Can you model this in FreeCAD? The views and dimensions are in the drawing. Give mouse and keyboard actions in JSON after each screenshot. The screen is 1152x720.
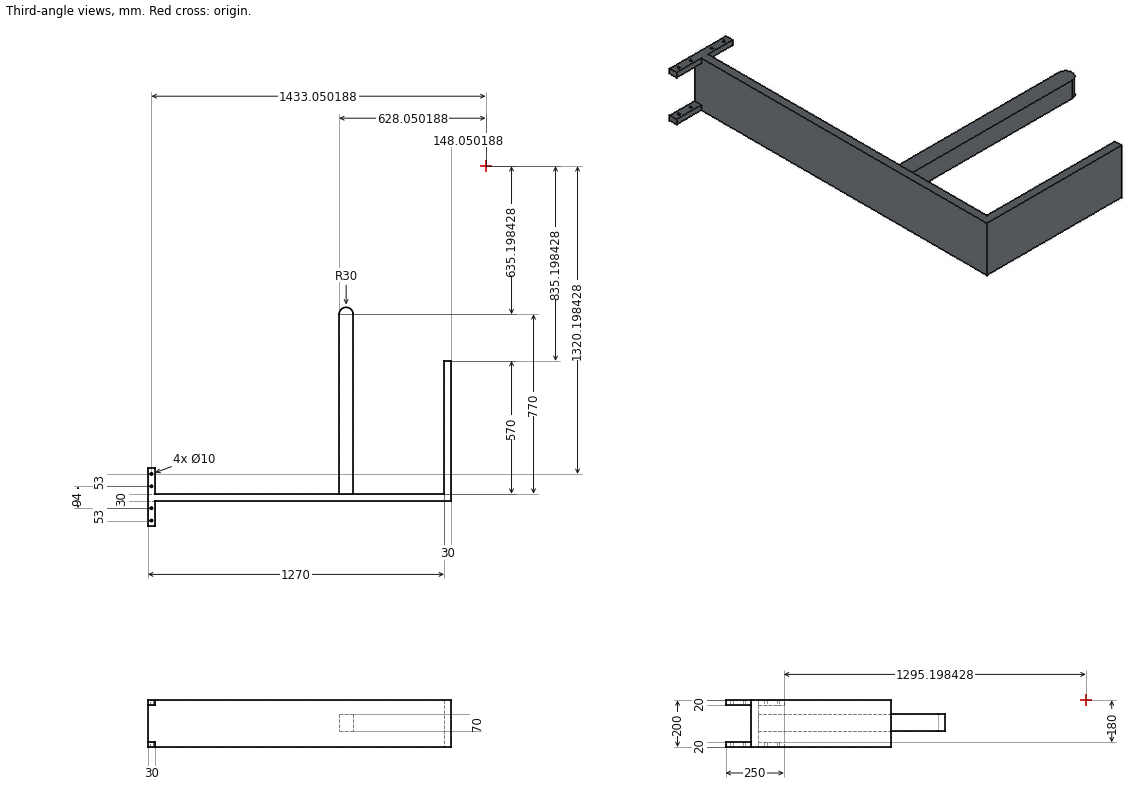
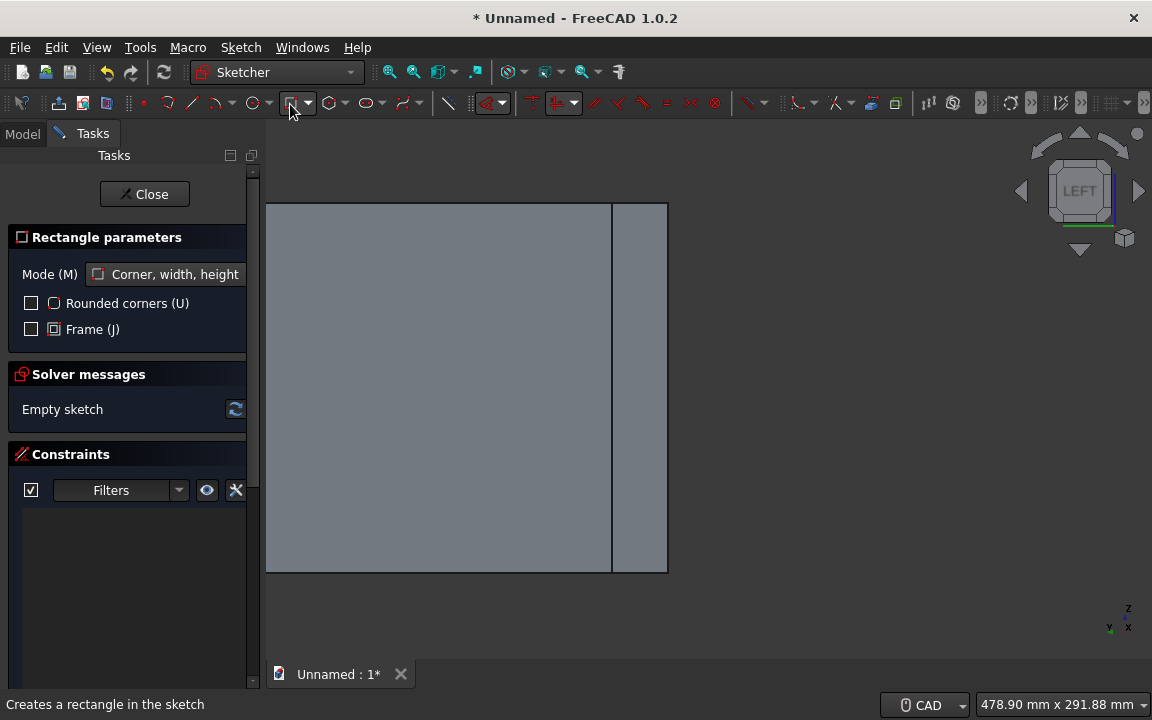
{"action": "left_click", "coordinate": [409, 536]}
{"action": "mouse_move", "coordinate": [871, 573]}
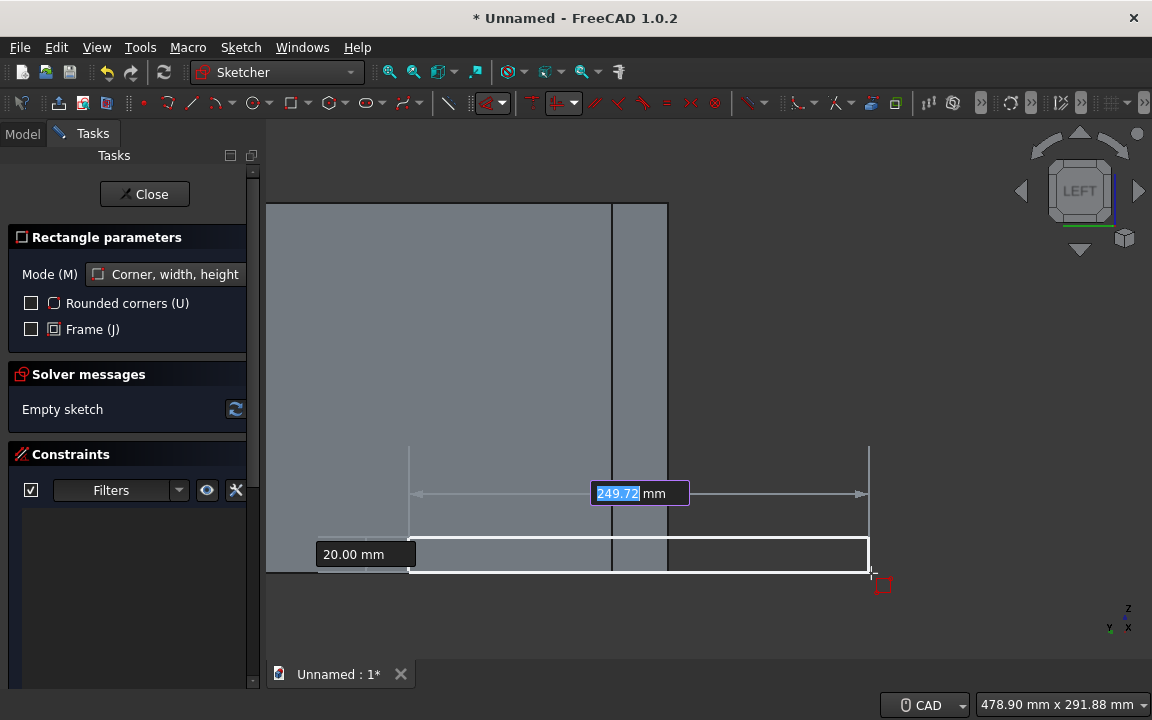
{"action": "type", "text": "250"}
{"action": "key", "text": "Tab"}
{"action": "type", "text": "20"}
{"action": "key", "text": "Return"}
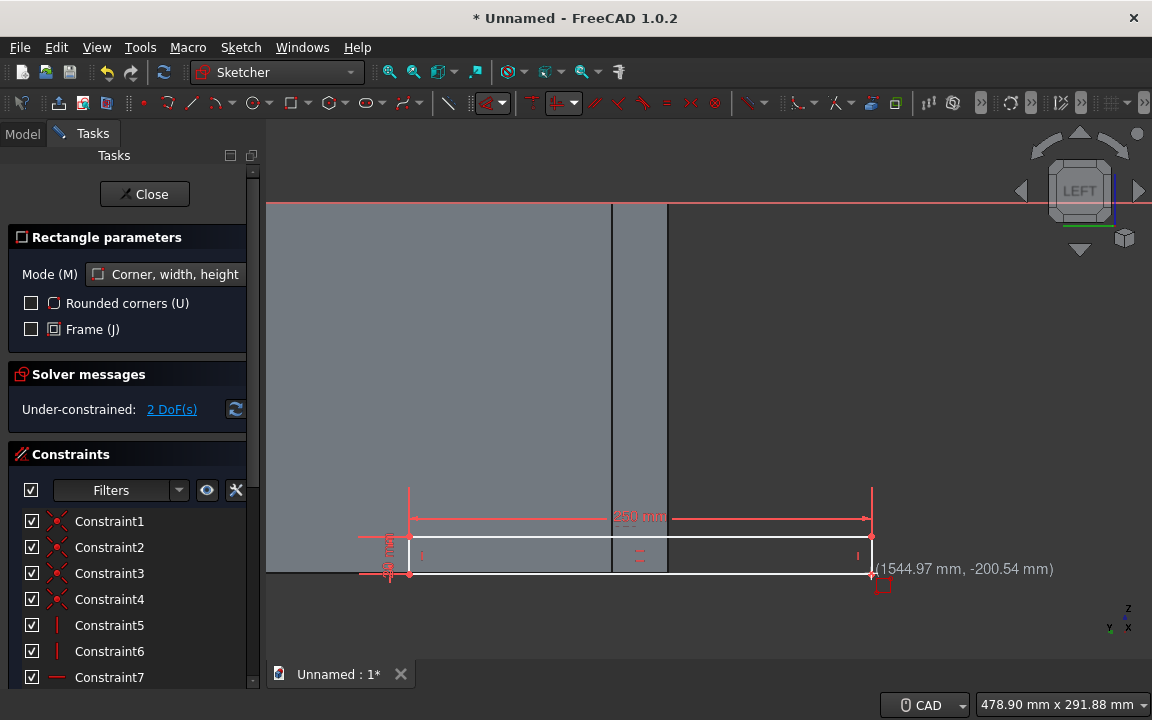
{"action": "left_click", "coordinate": [409, 203]}
{"action": "mouse_move", "coordinate": [871, 240]}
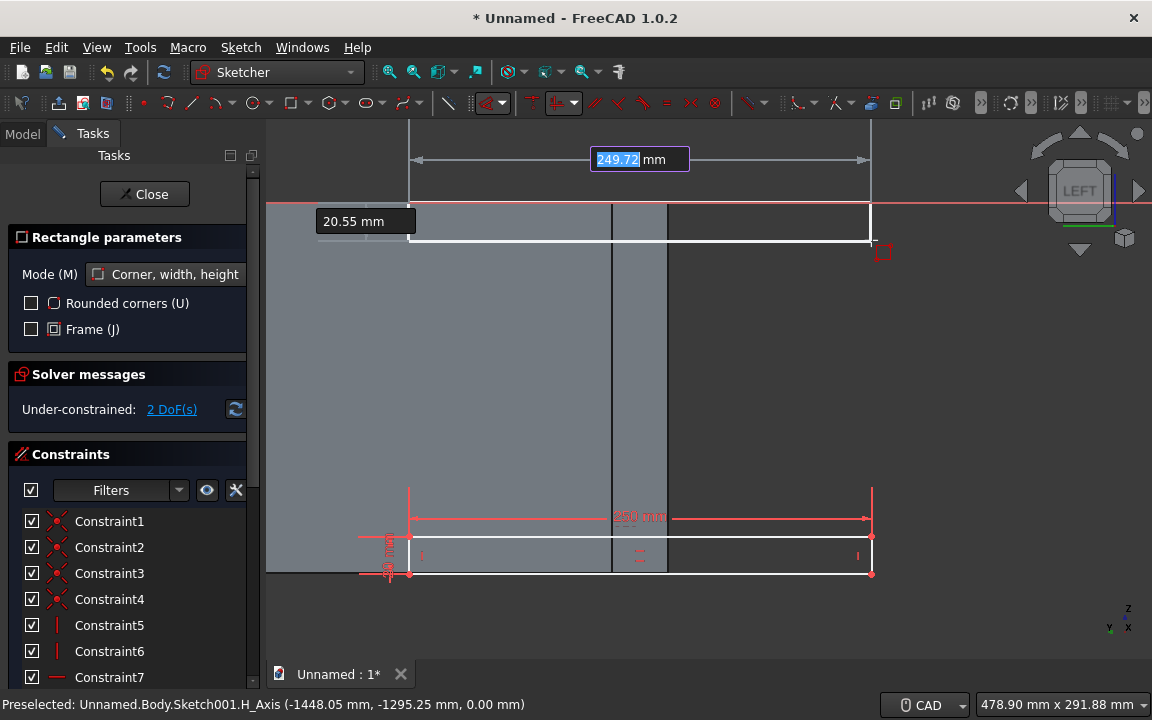
{"action": "type", "text": "250"}
{"action": "key", "text": "Tab"}
{"action": "type", "text": "20"}
{"action": "key", "text": "Return"}
{"action": "key", "text": "Escape"}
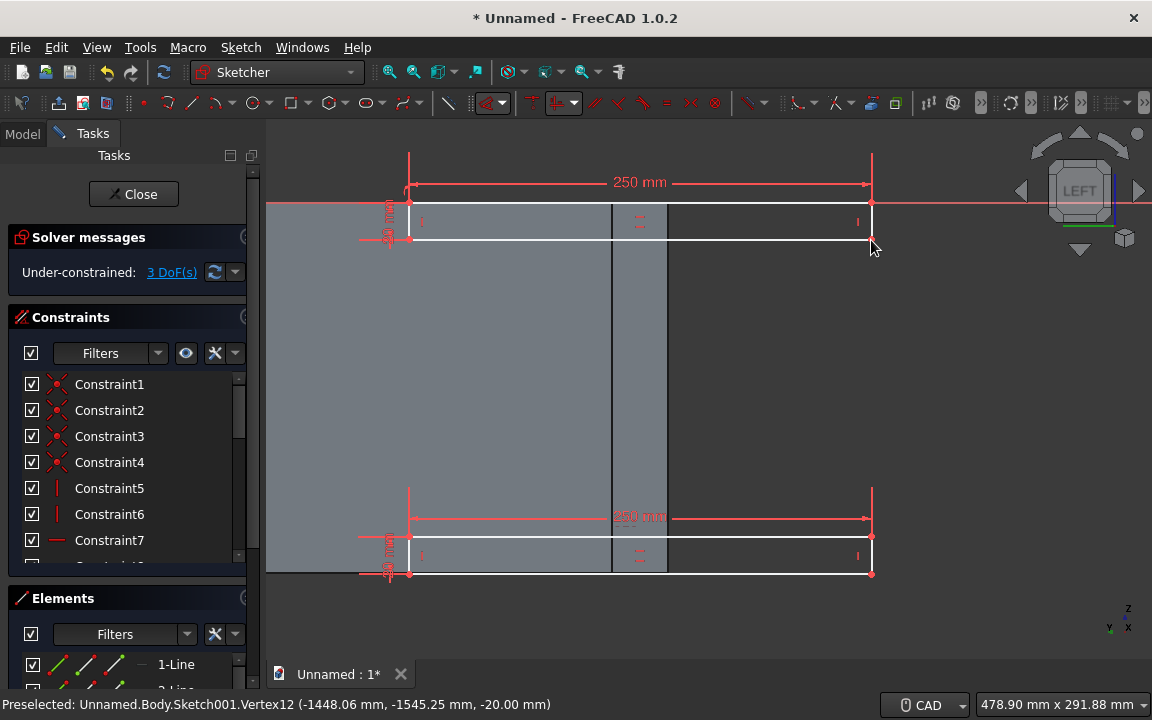
{"action": "left_click", "coordinate": [409, 537]}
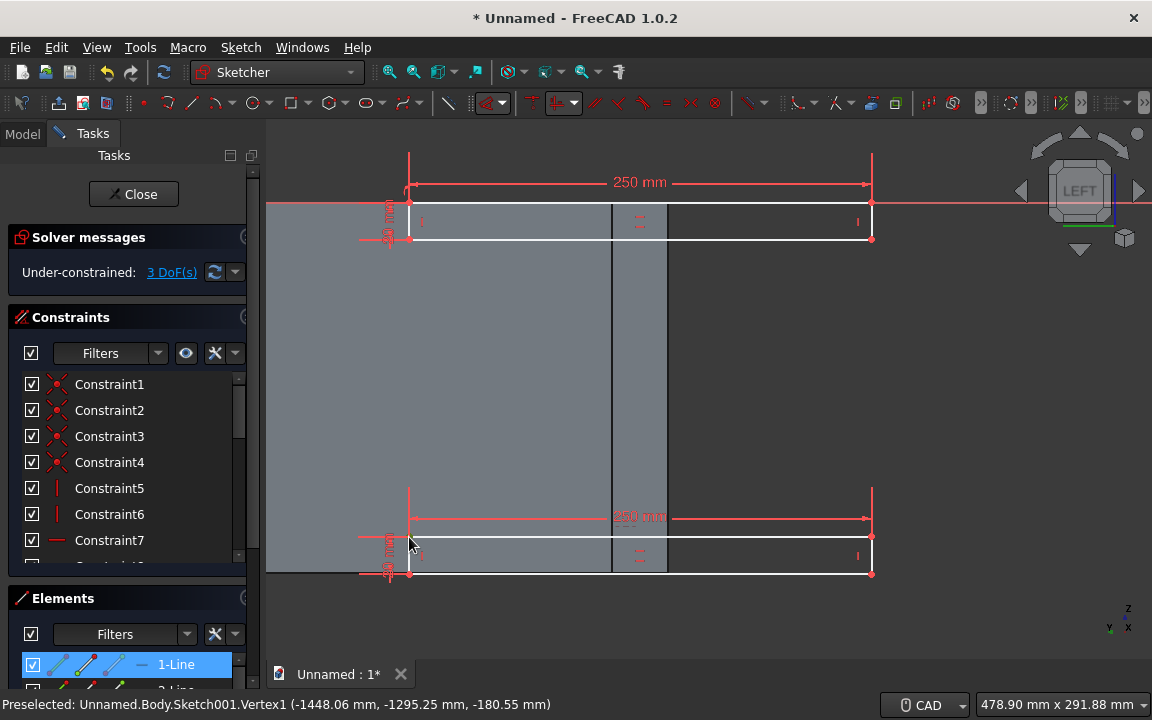
{"action": "key", "text": "i"}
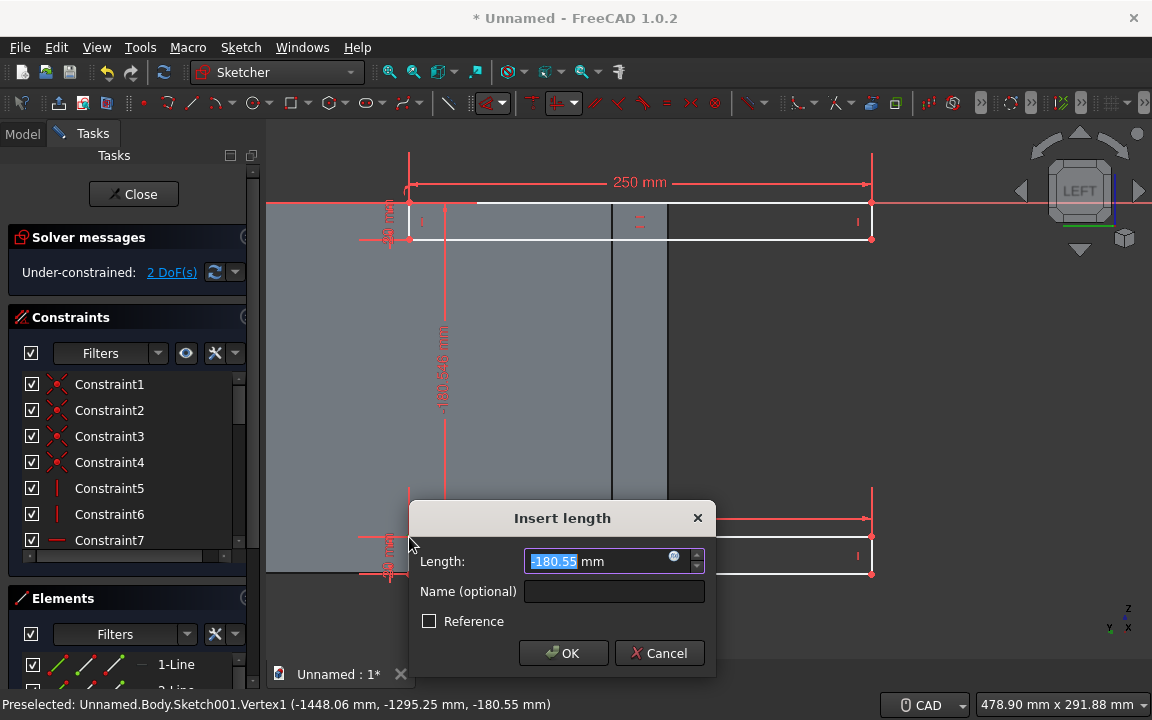
{"action": "type", "text": "-180"}
{"action": "key", "text": "Return"}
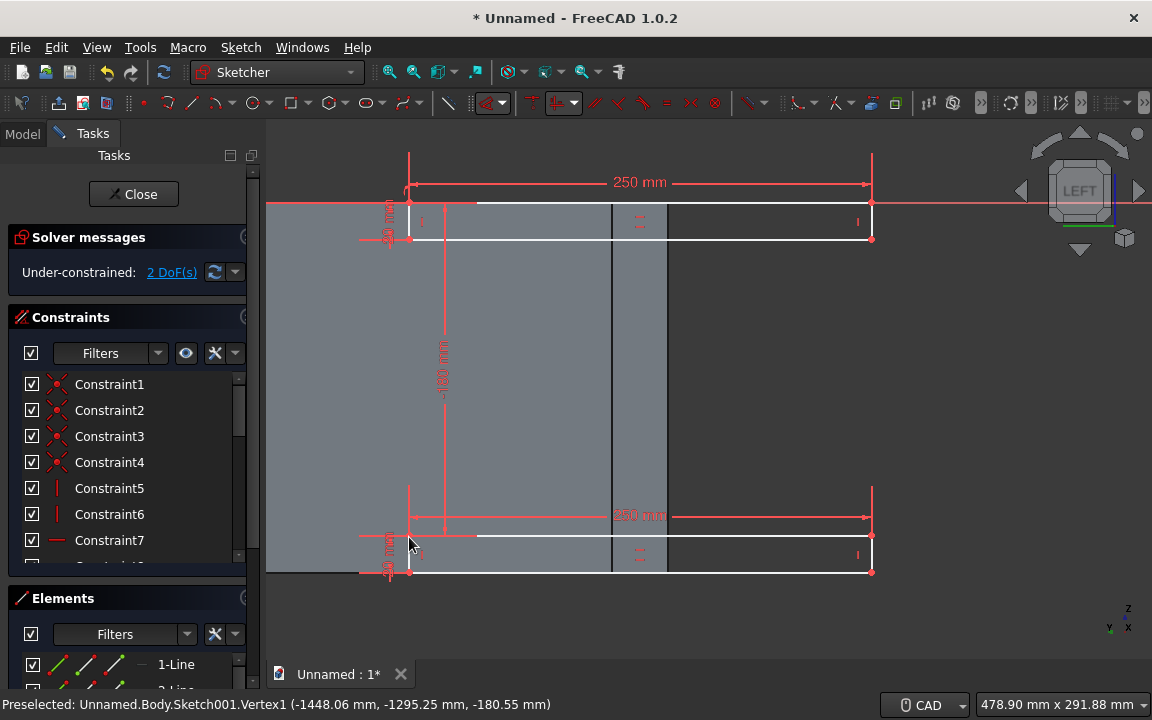
{"action": "left_click", "coordinate": [409, 536]}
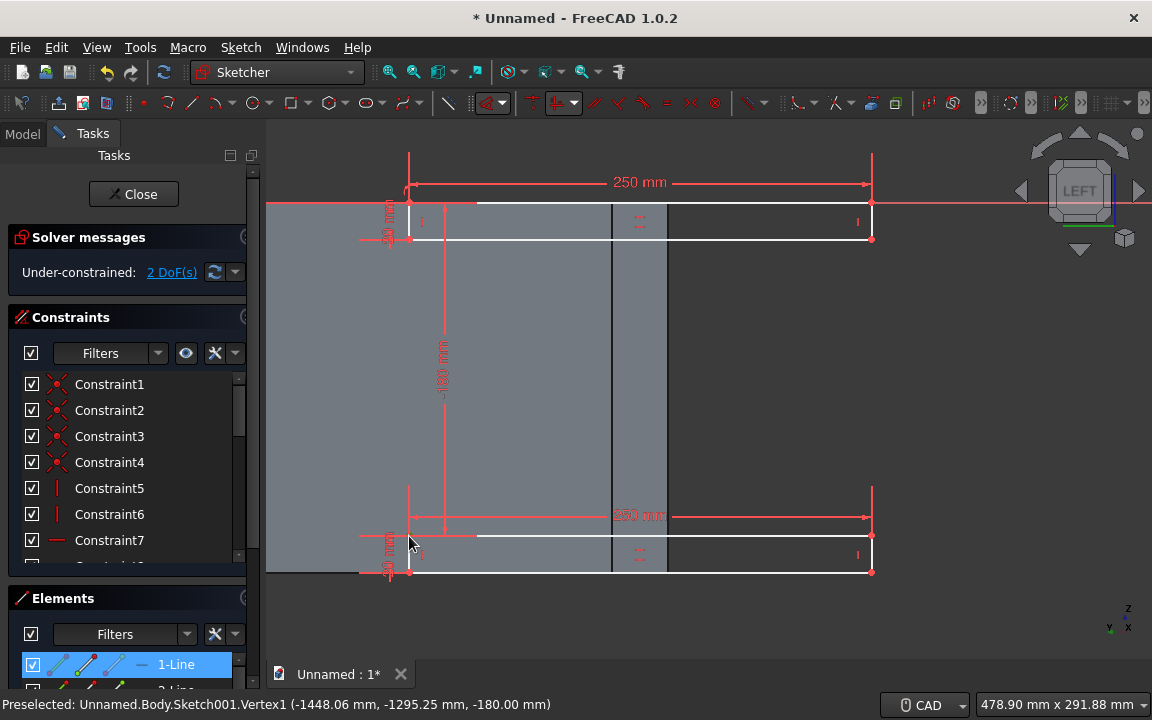
{"action": "left_click", "coordinate": [504, 104]}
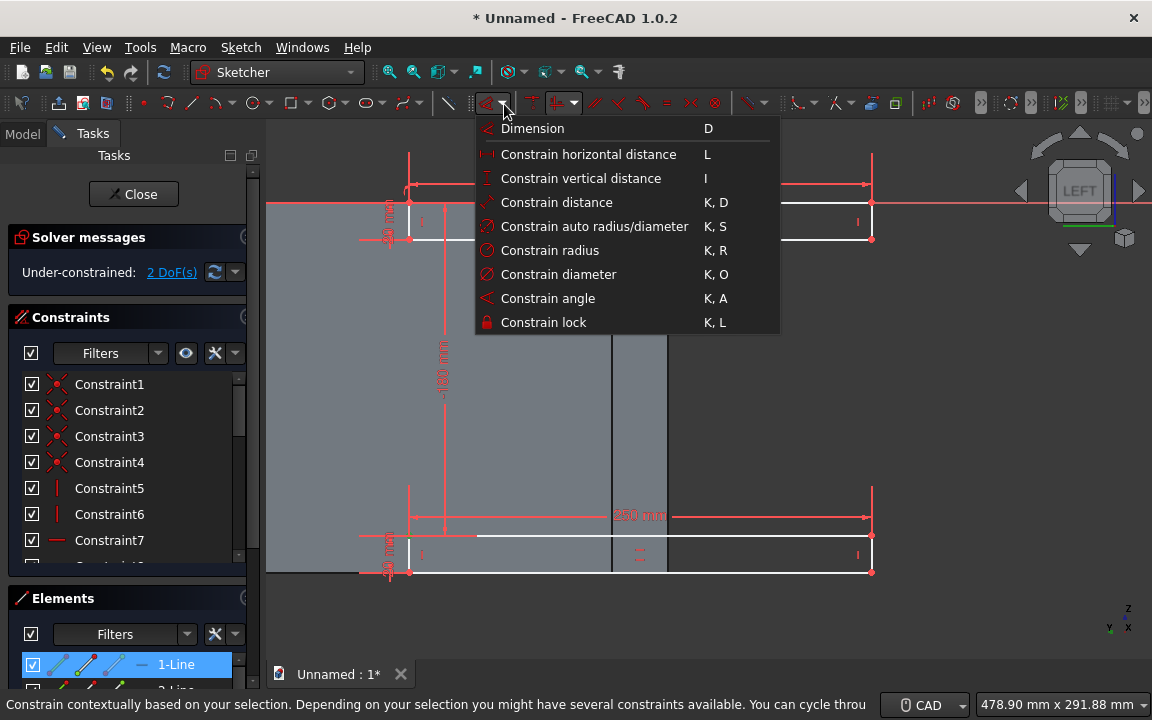
{"action": "left_click", "coordinate": [628, 154]}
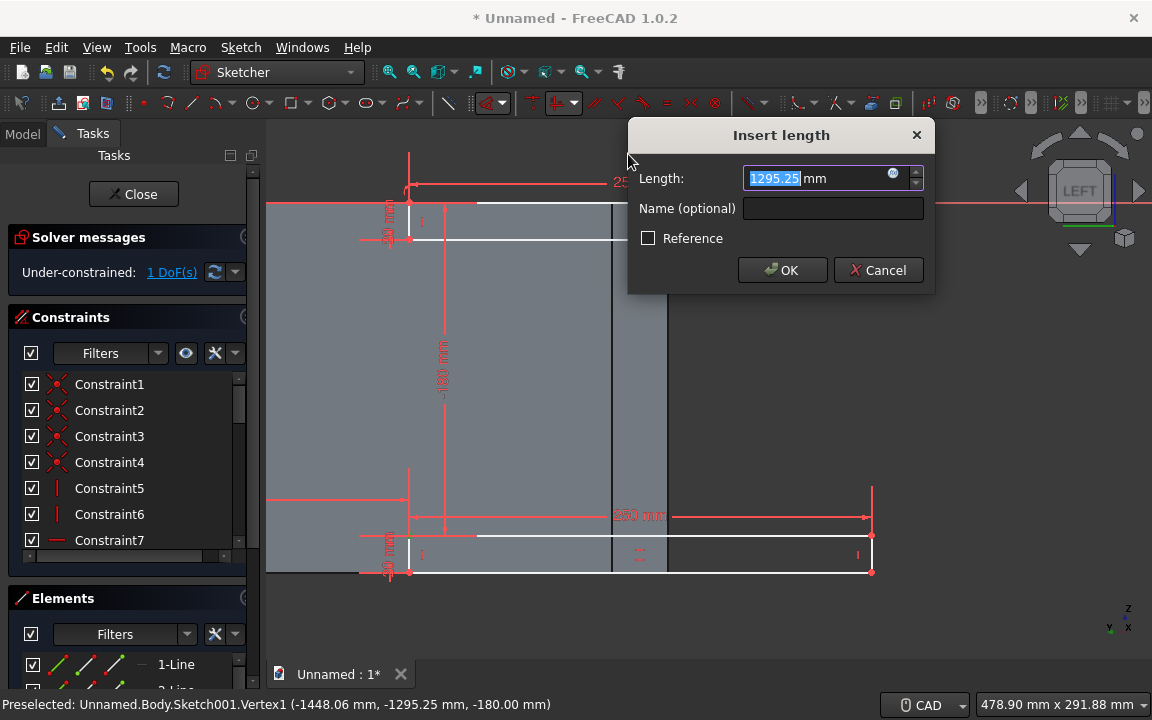
{"action": "type", "text": "1295.198428"}
{"action": "key", "text": "Return"}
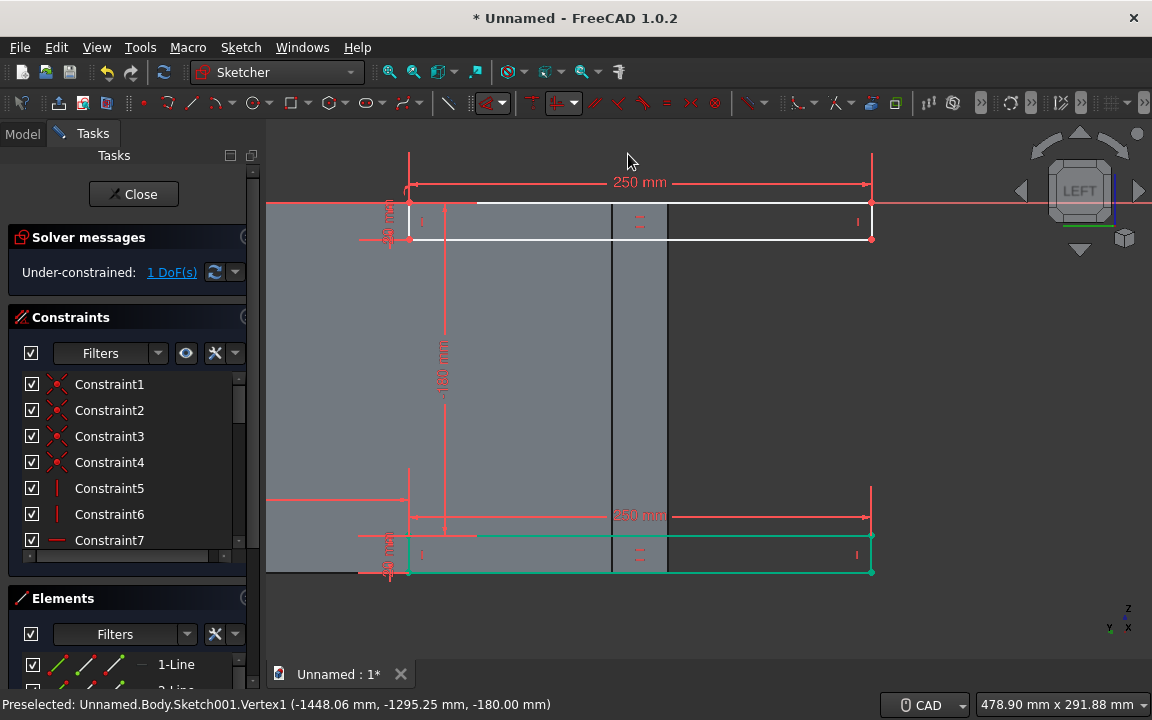
{"action": "left_click", "coordinate": [409, 203]}